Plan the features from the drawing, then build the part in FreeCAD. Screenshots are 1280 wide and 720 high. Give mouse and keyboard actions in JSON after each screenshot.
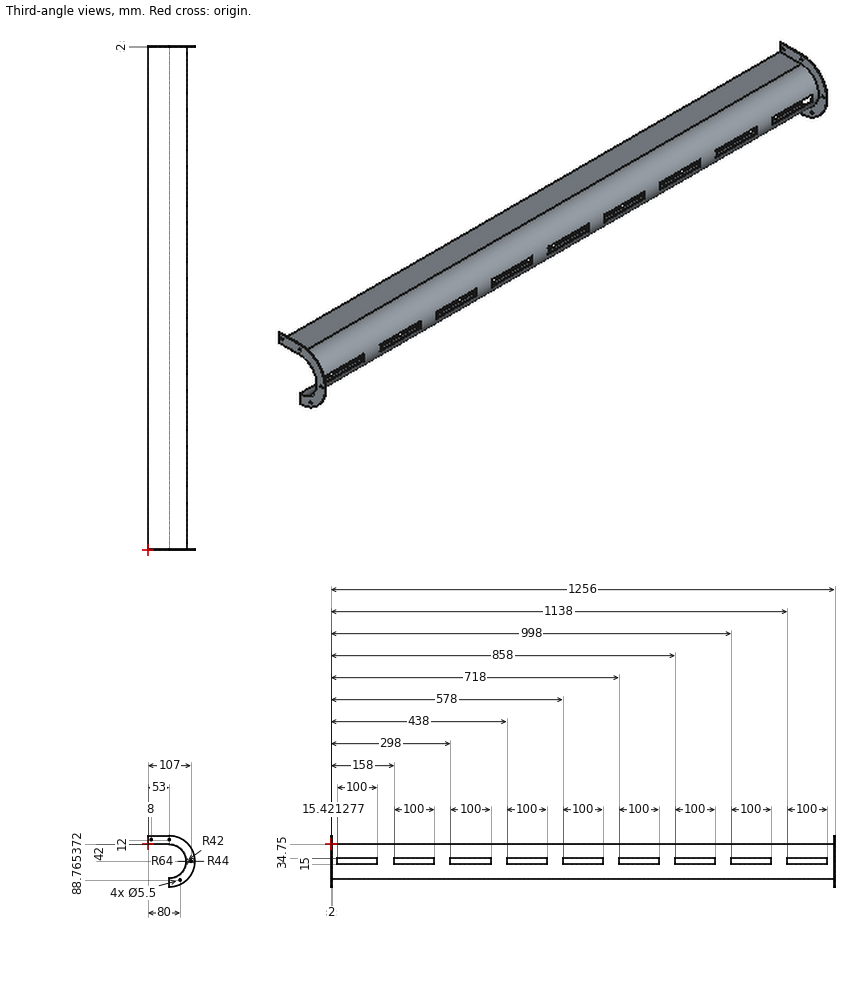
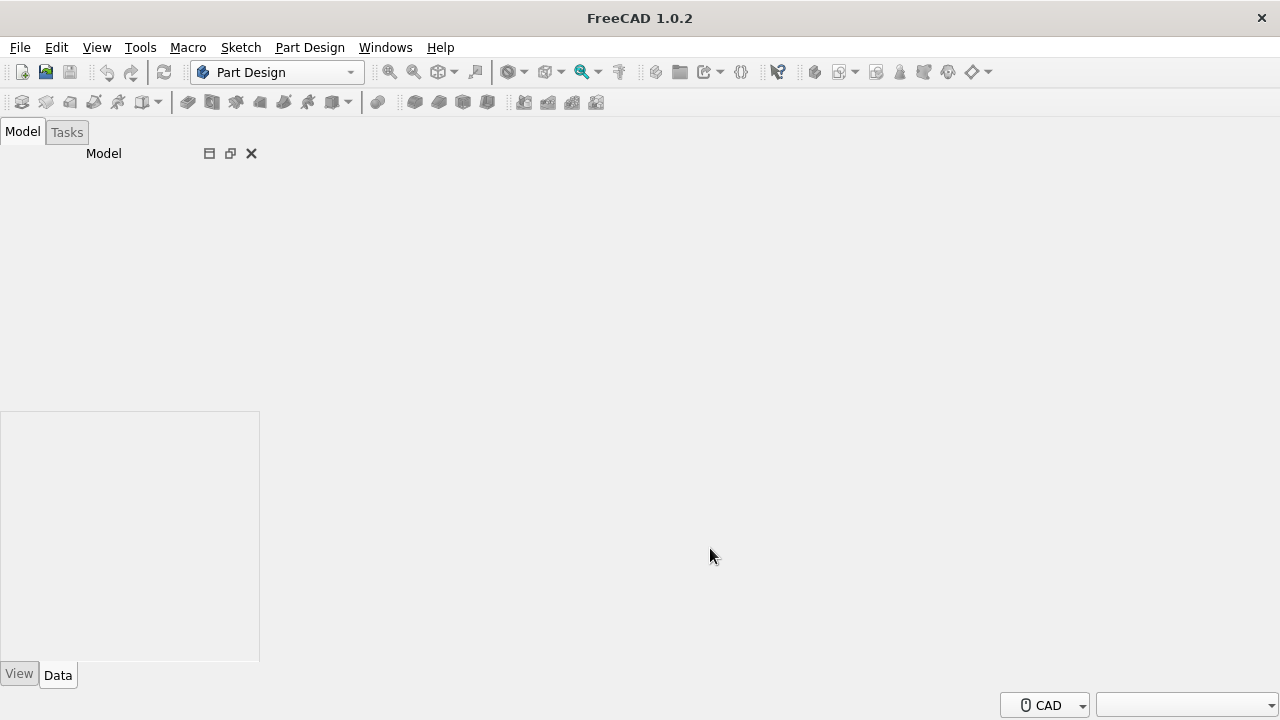
{"action": "key", "text": "ctrl+n"}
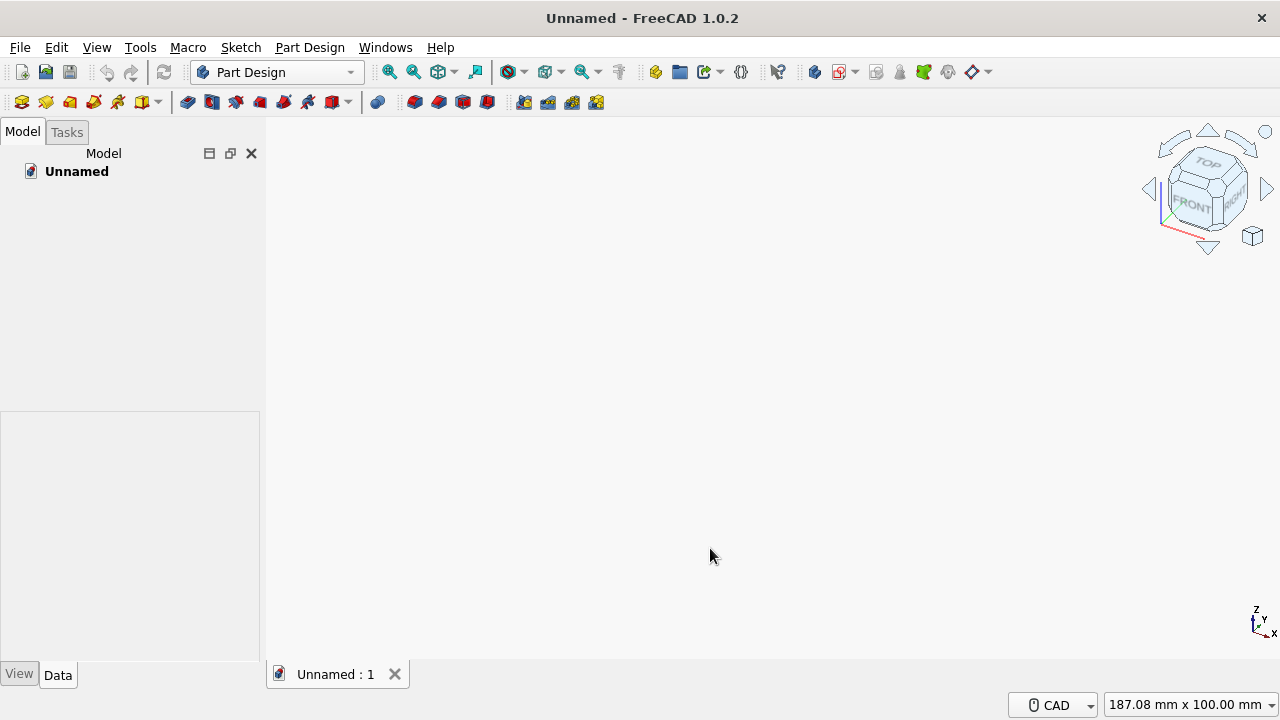
{"action": "left_click", "coordinate": [840, 72]}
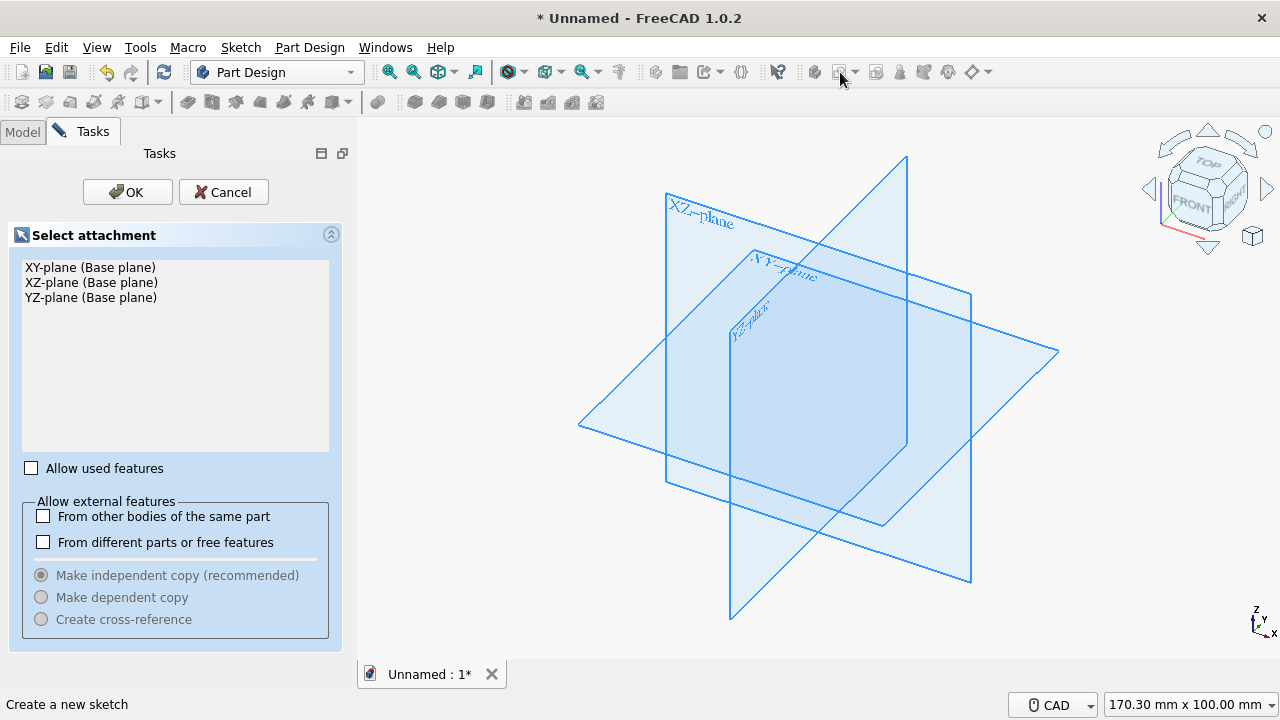
{"action": "left_click", "coordinate": [82, 282]}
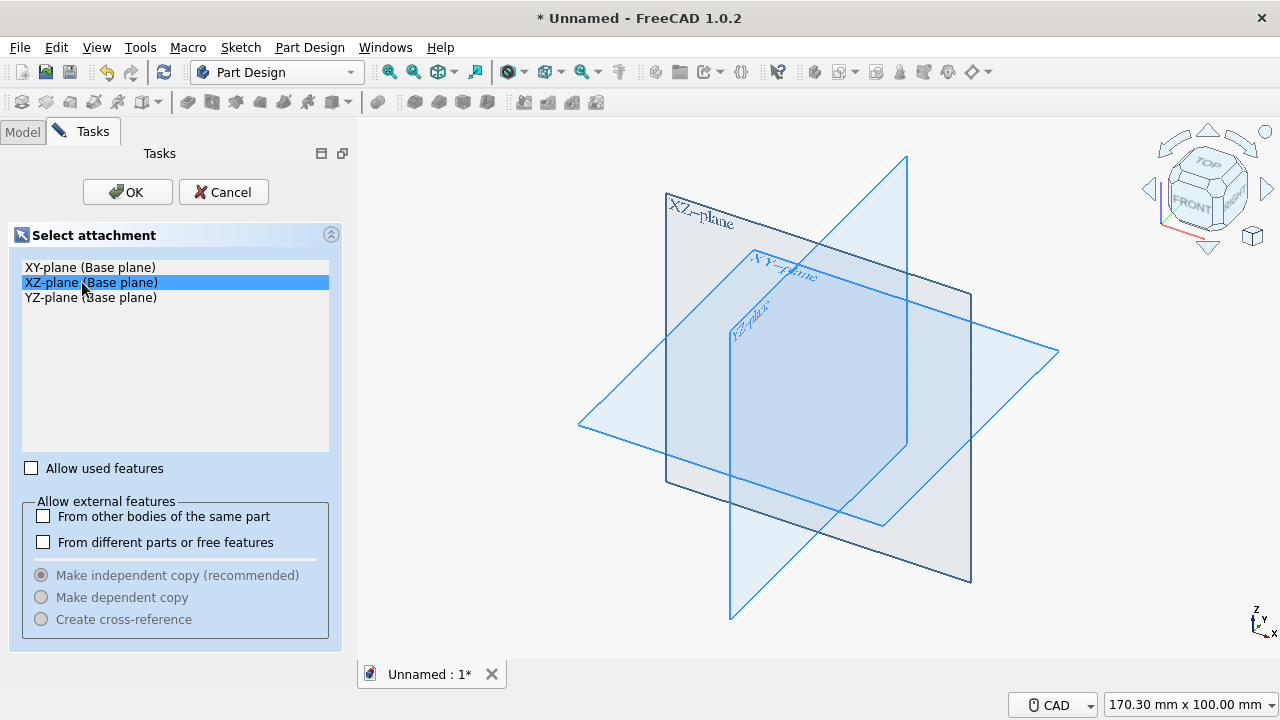
{"action": "left_click", "coordinate": [128, 192]}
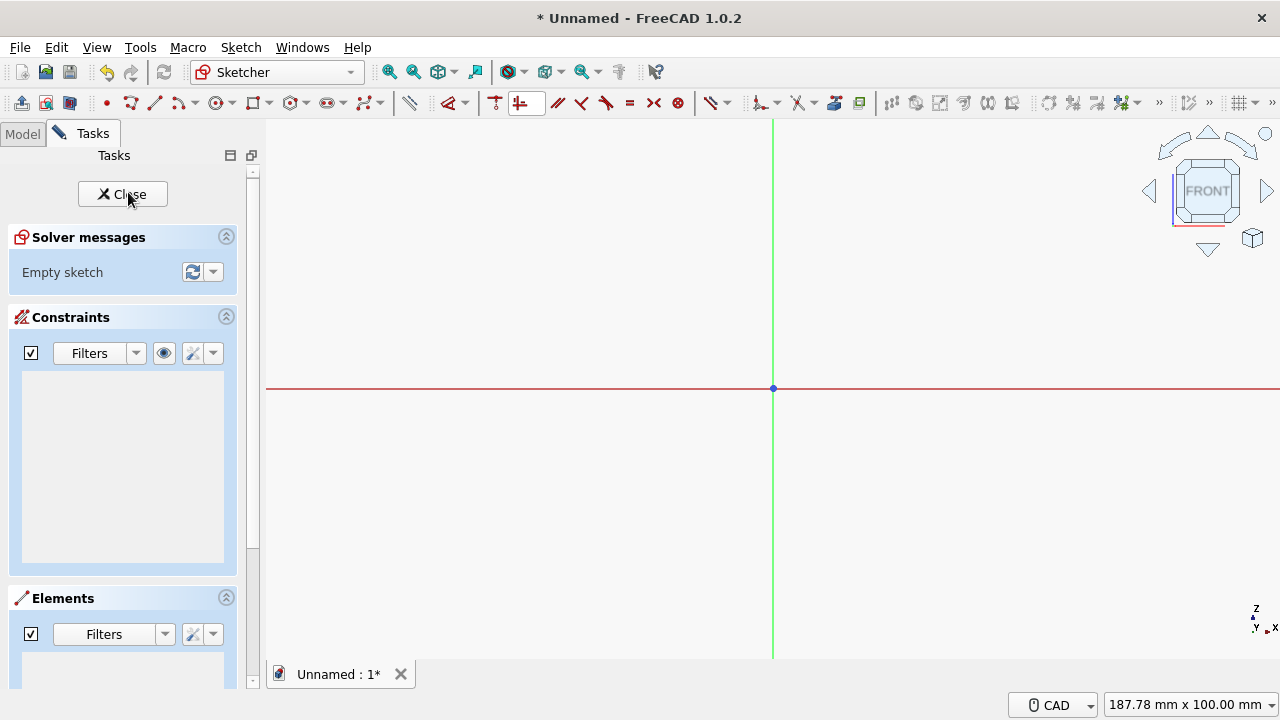
{"action": "scroll", "coordinate": [303, 147], "scroll_direction": "down", "scroll_amount": 3}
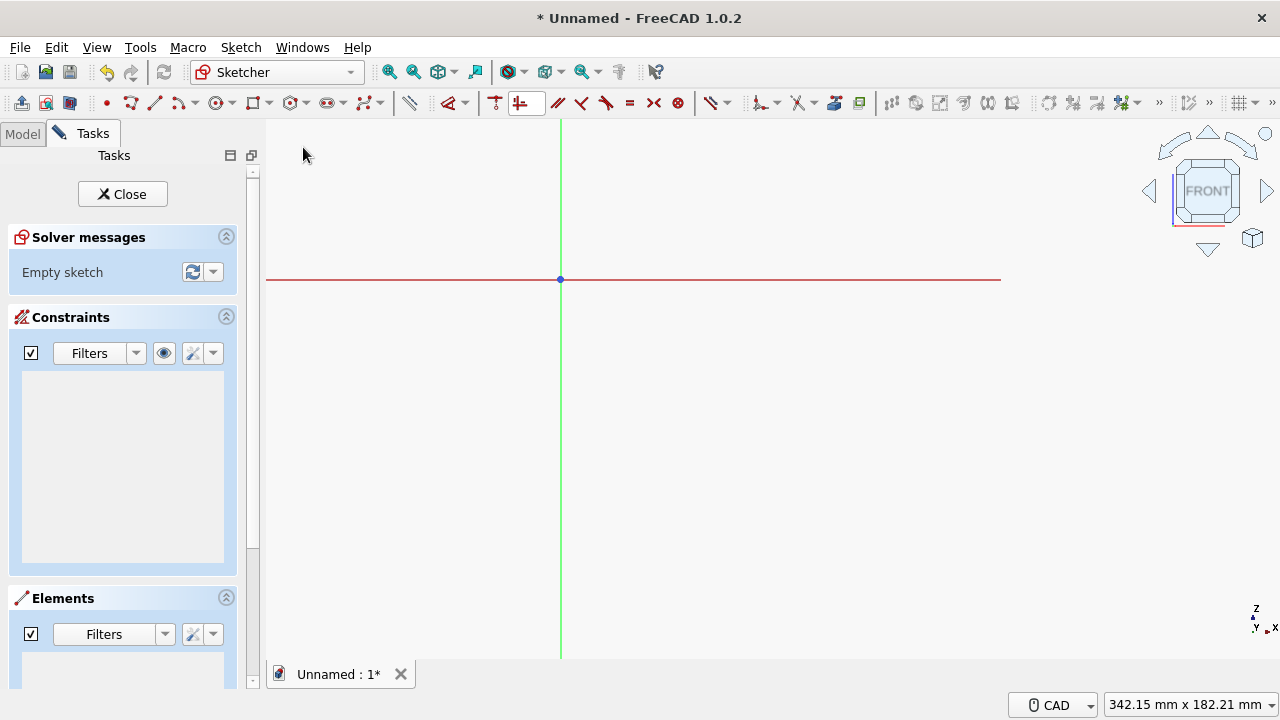
{"action": "left_click", "coordinate": [132, 104]}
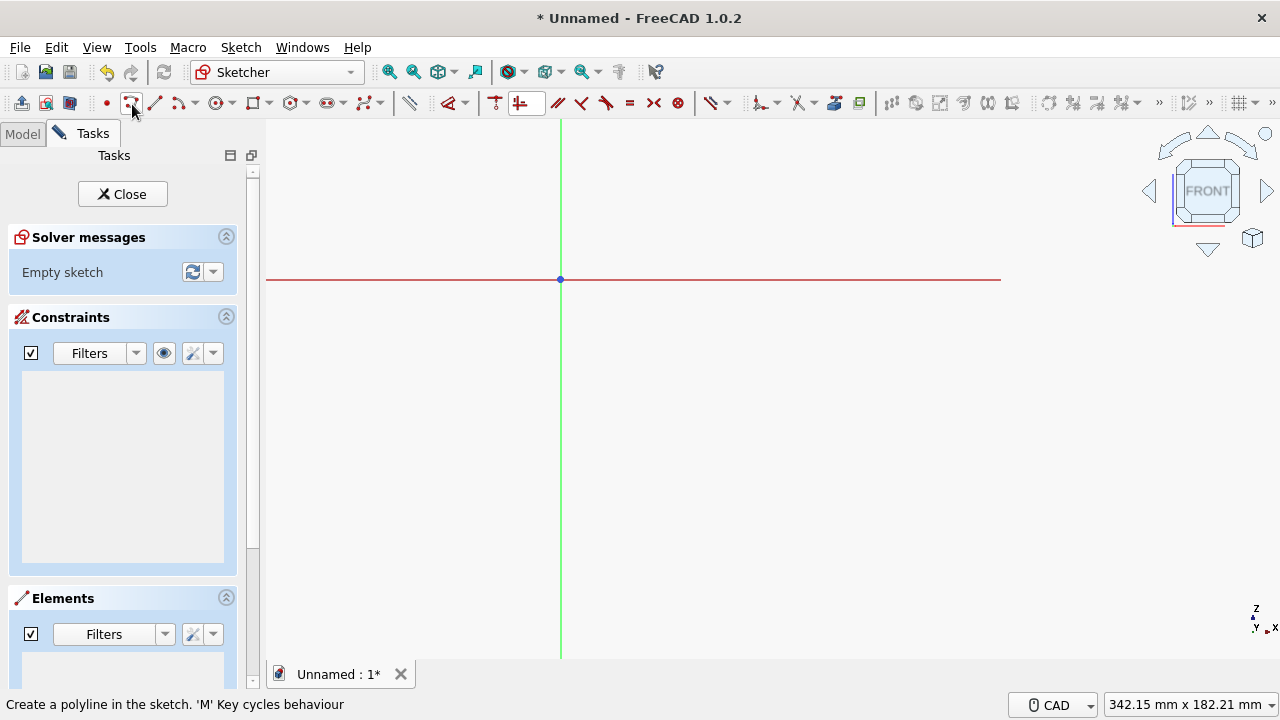
{"action": "left_click", "coordinate": [718, 280]}
{"action": "left_click", "coordinate": [561, 280]}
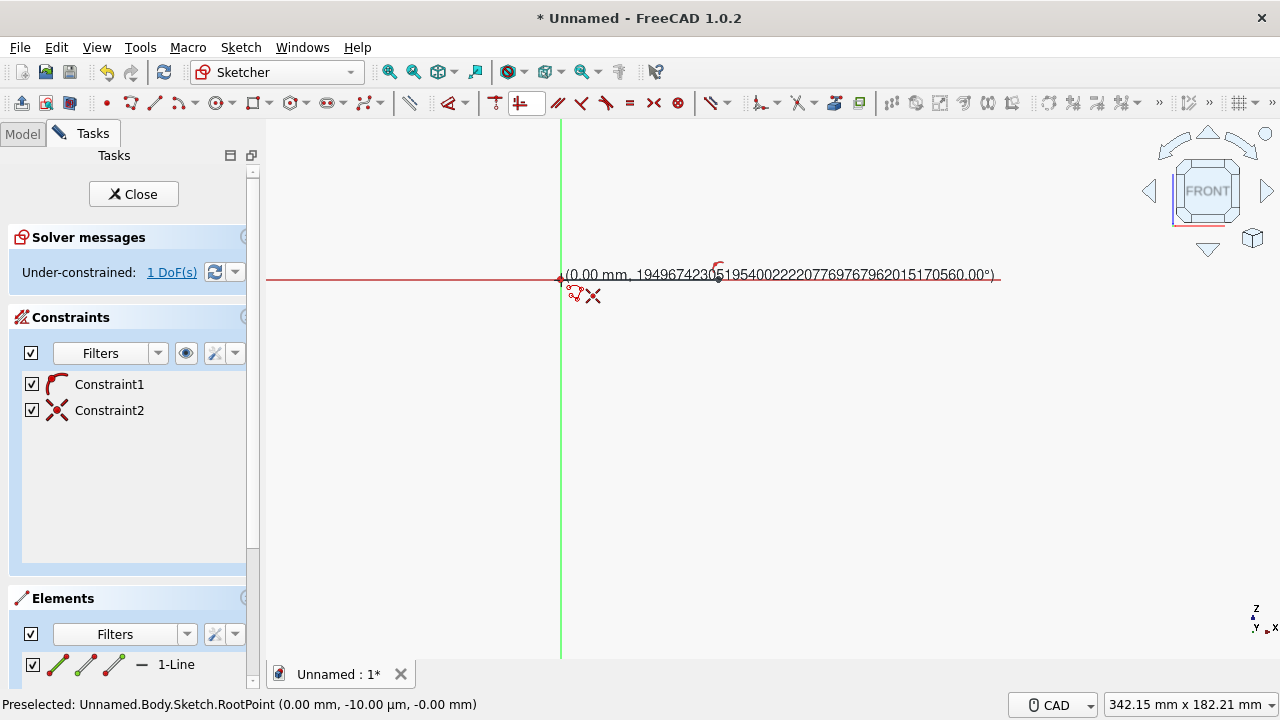
{"action": "scroll", "coordinate": [561, 274], "scroll_direction": "up", "scroll_amount": 5}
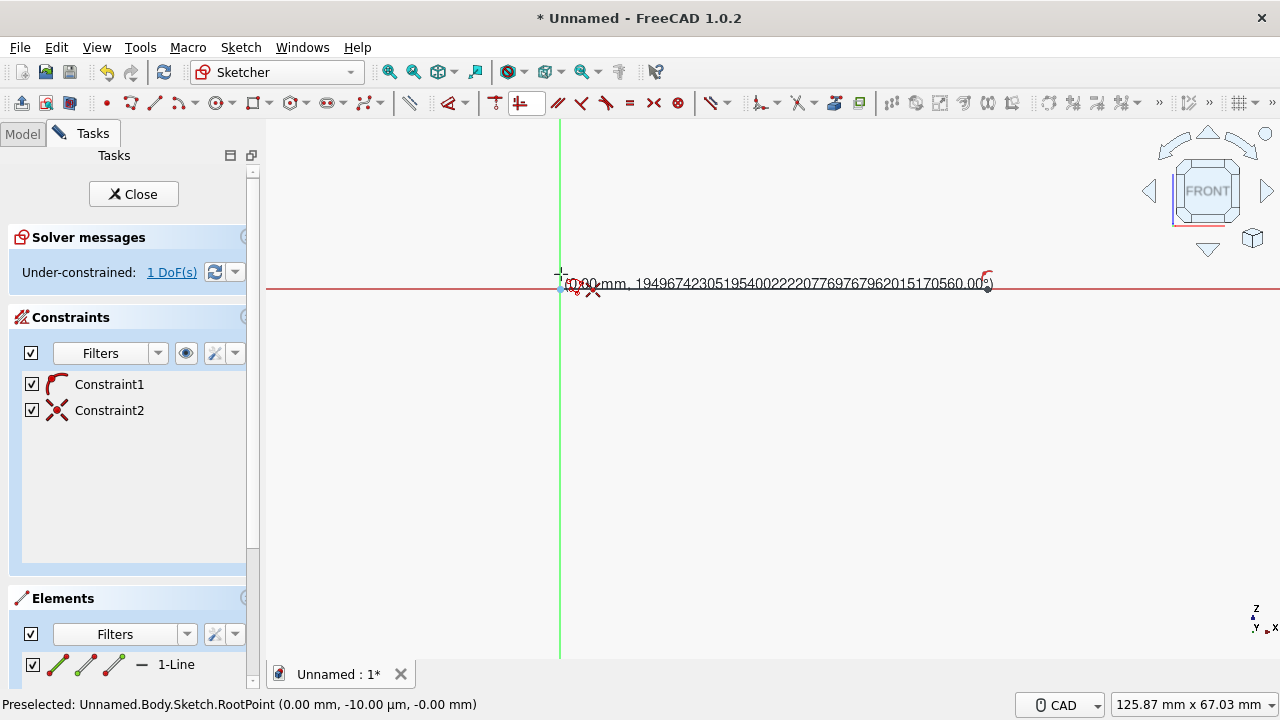
{"action": "left_click", "coordinate": [569, 273]}
{"action": "left_click", "coordinate": [987, 273]}
{"action": "right_click", "coordinate": [987, 273]}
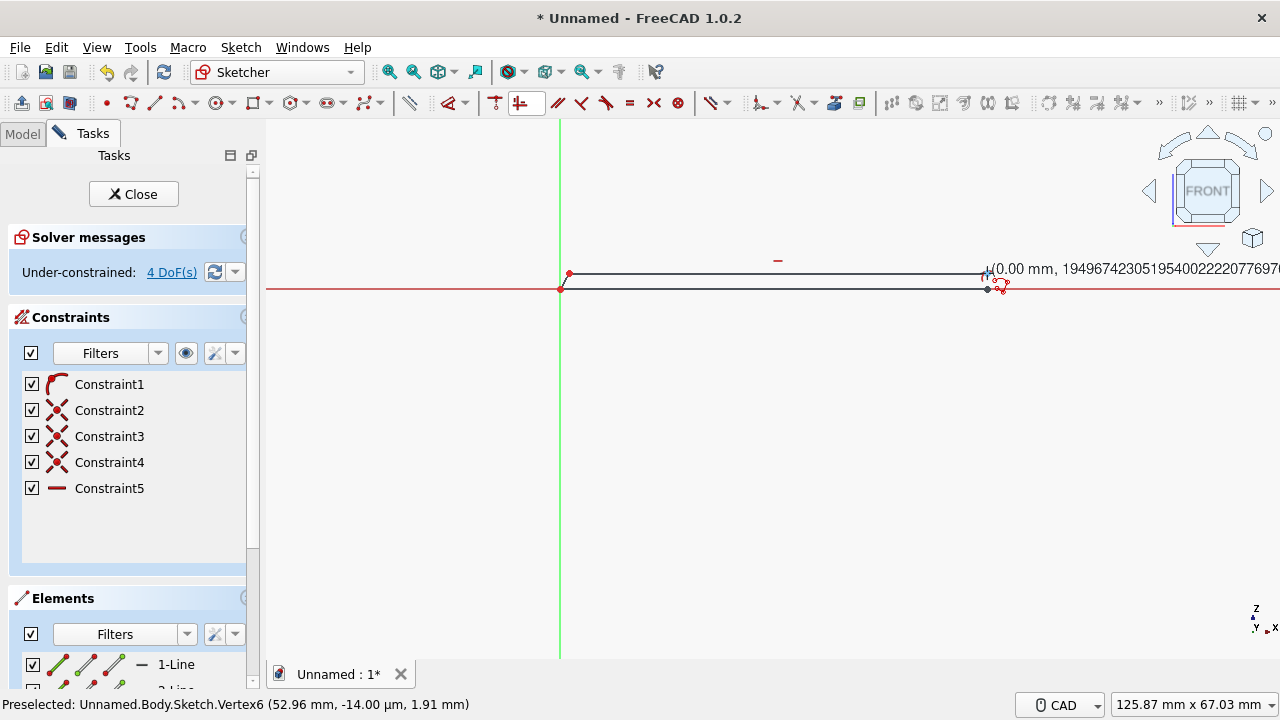
{"action": "left_click", "coordinate": [156, 104]}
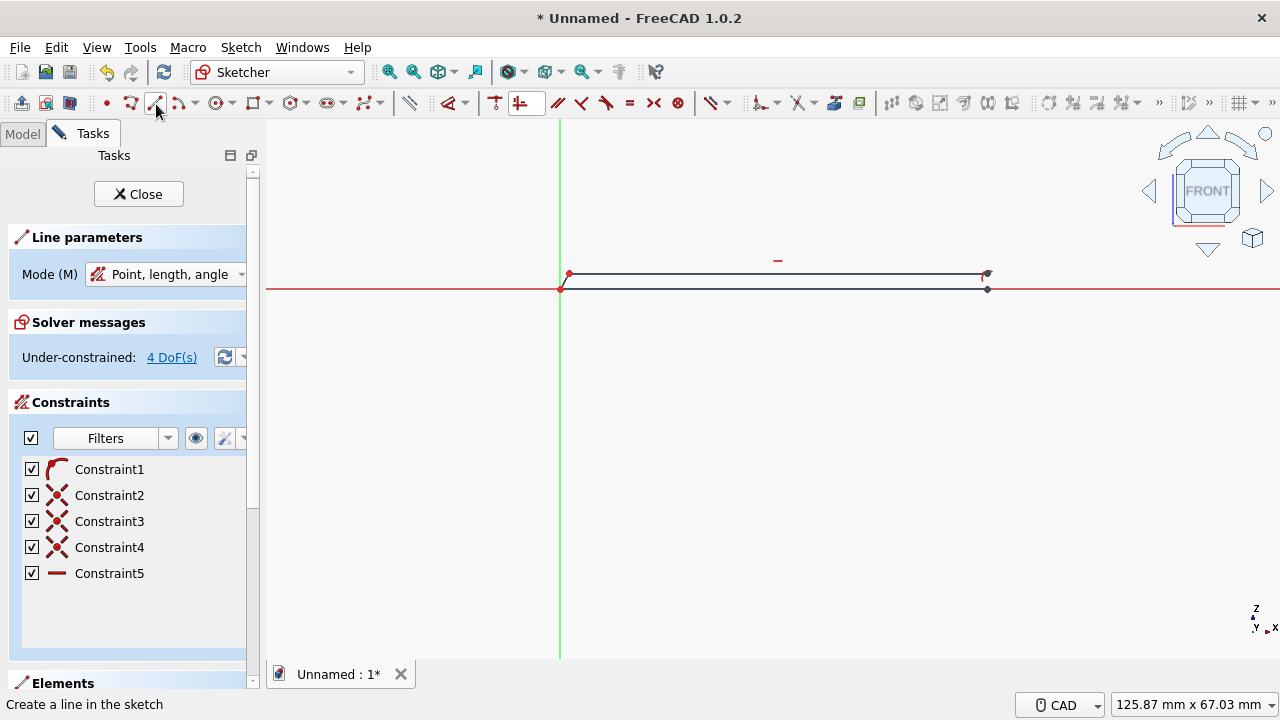
{"action": "scroll", "coordinate": [503, 194], "scroll_direction": "down", "scroll_amount": 4}